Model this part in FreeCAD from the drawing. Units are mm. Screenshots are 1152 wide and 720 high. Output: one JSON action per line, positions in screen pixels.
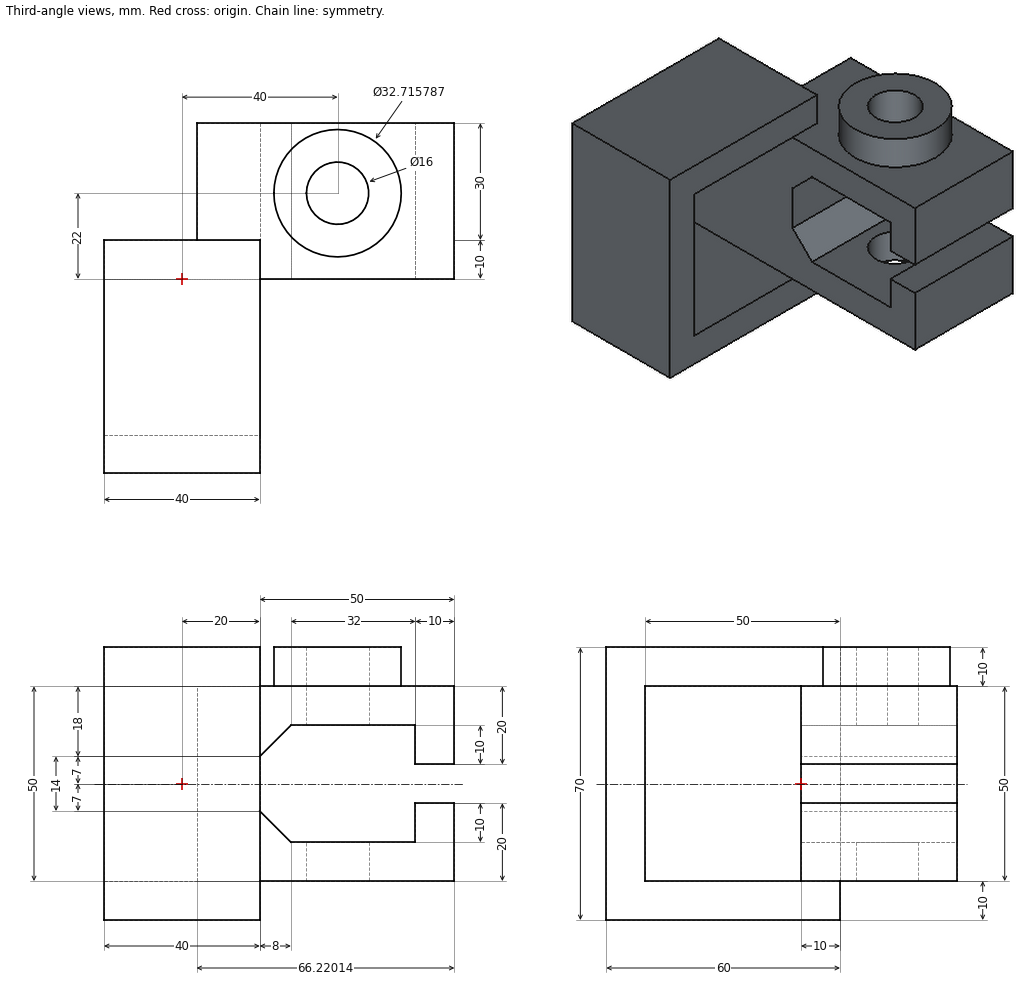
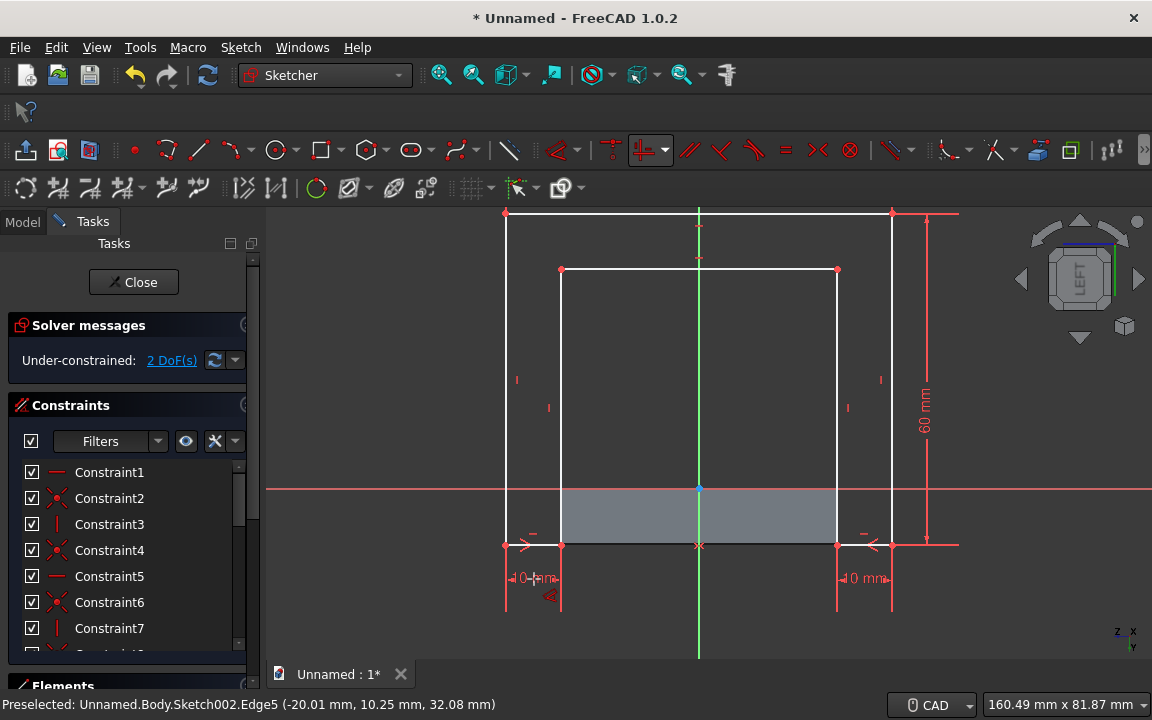
{"action": "left_click", "coordinate": [561, 462]}
{"action": "left_click", "coordinate": [527, 407]}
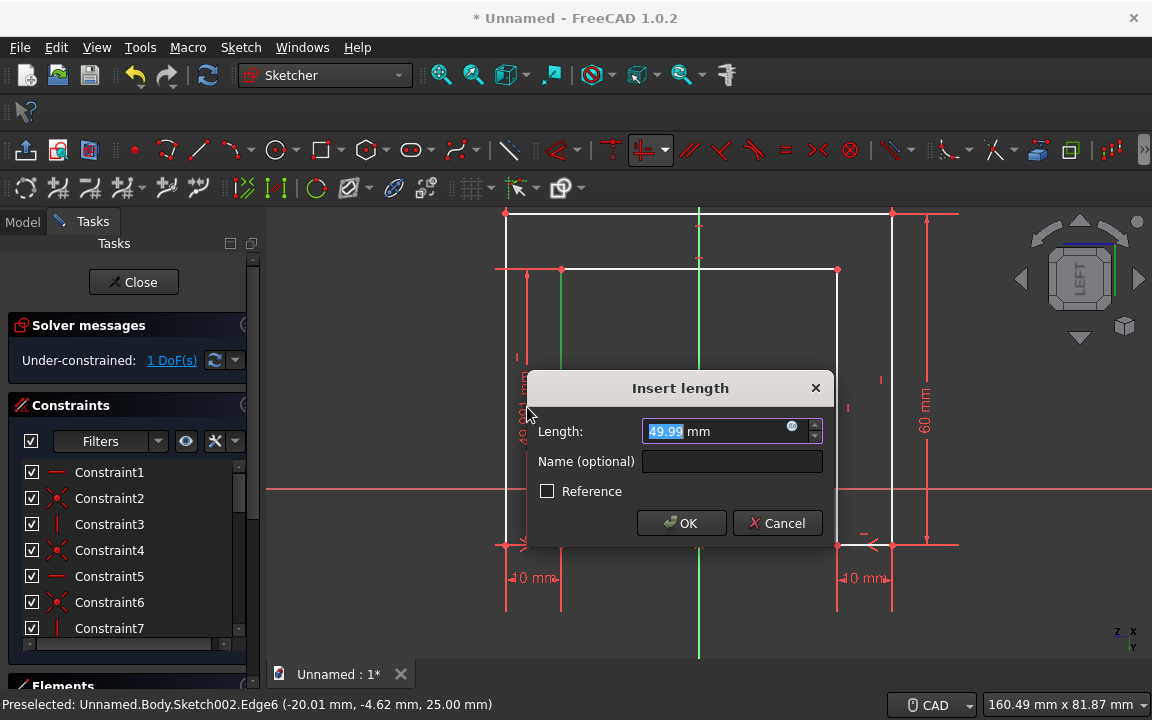
{"action": "type", "text": "50"}
{"action": "key", "text": "Return"}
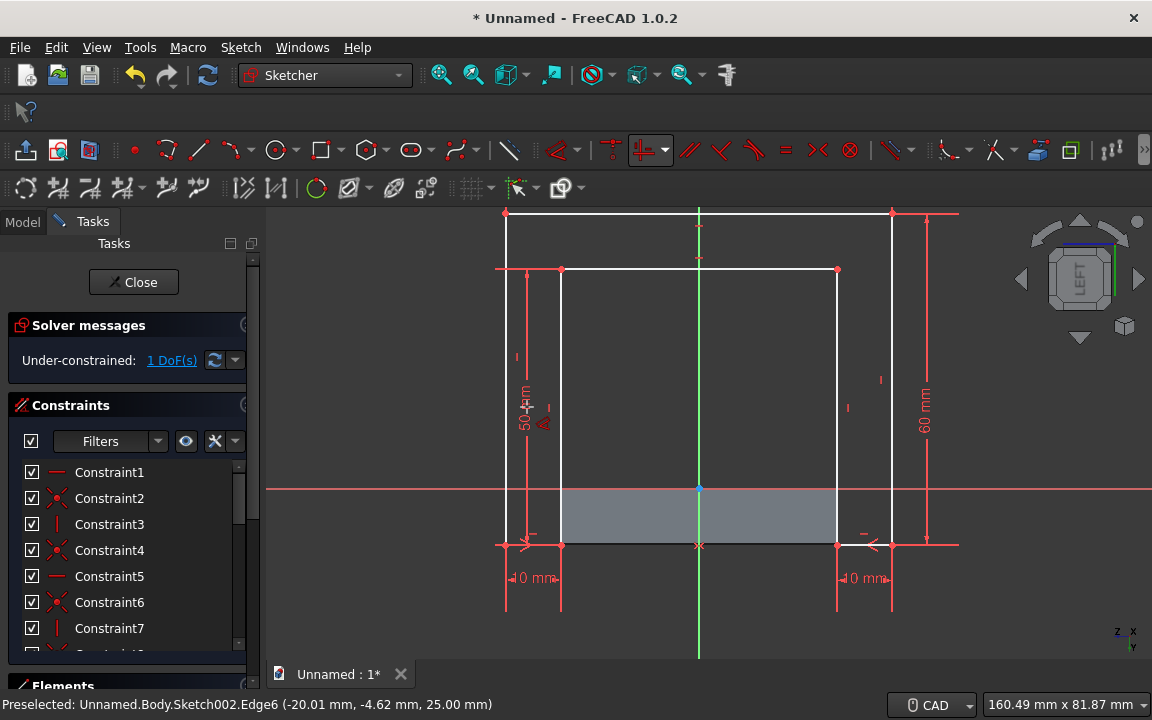
{"action": "left_click", "coordinate": [837, 545]}
{"action": "left_click", "coordinate": [871, 517]}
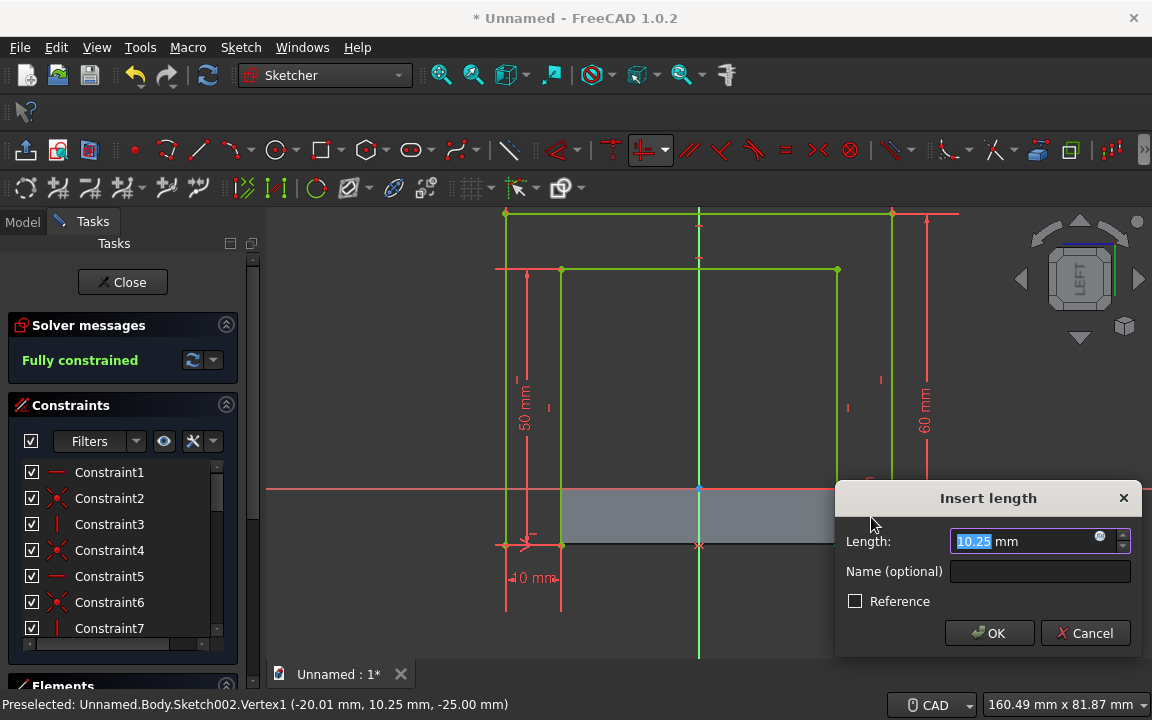
{"action": "type", "text": "10"}
{"action": "key", "text": "Return"}
{"action": "key", "text": "Escape"}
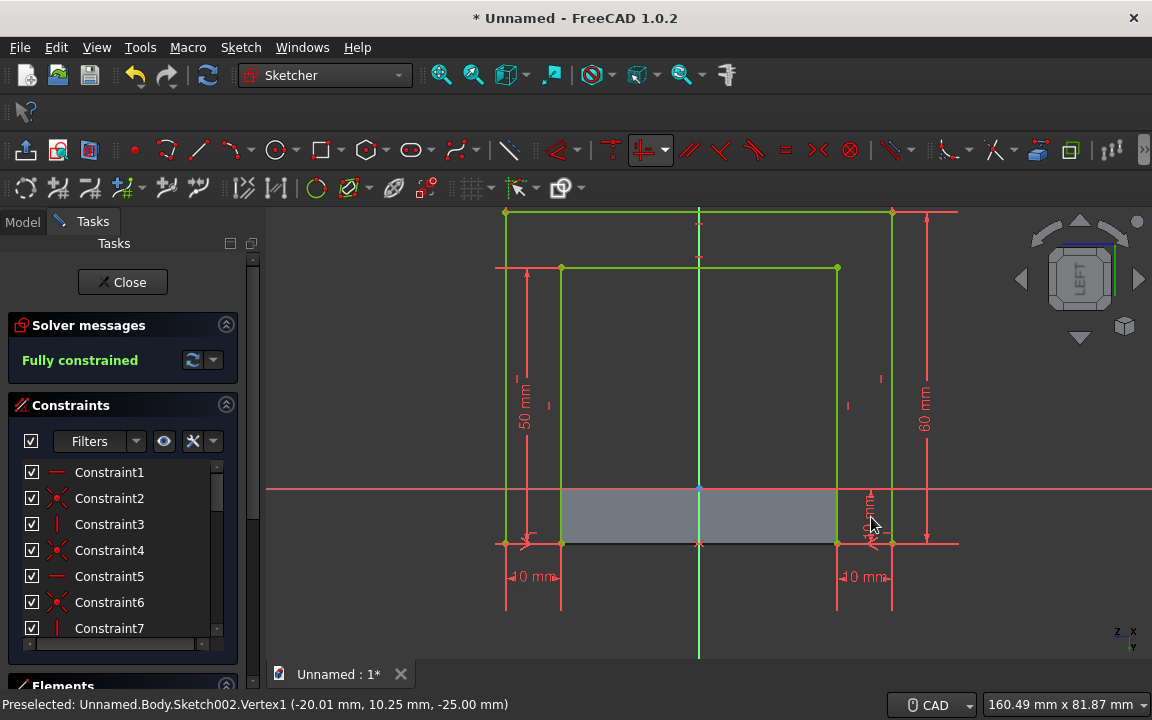
{"action": "left_click", "coordinate": [123, 282]}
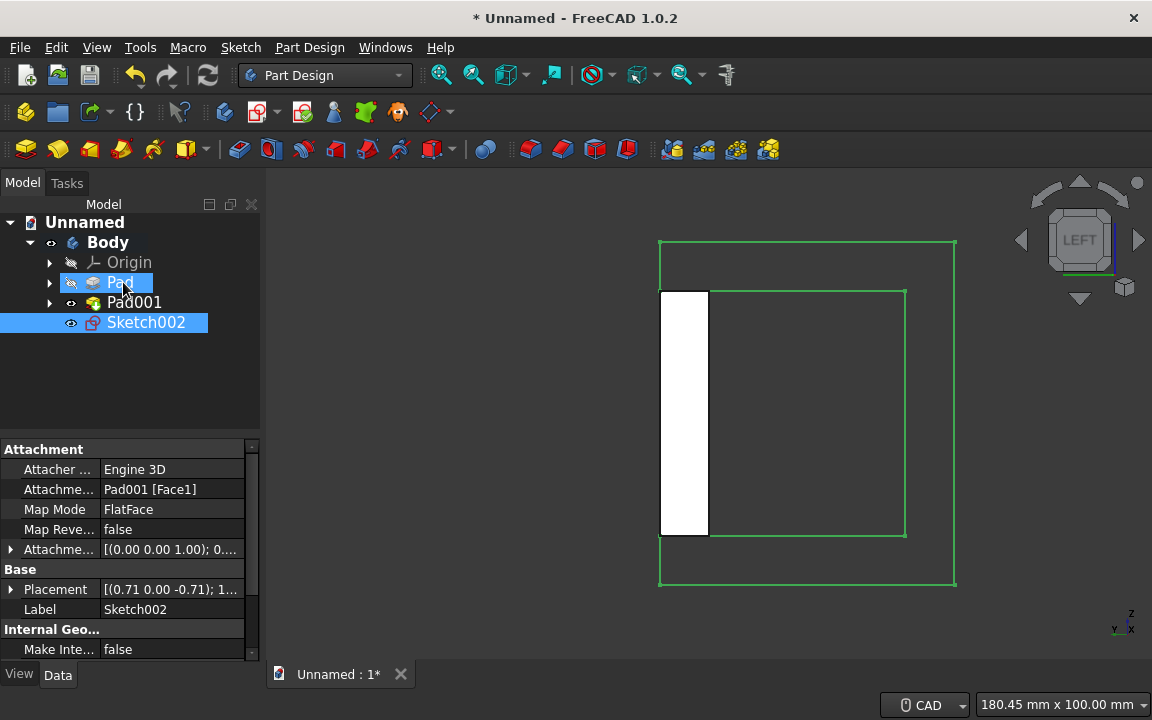
{"action": "left_click", "coordinate": [26, 150]}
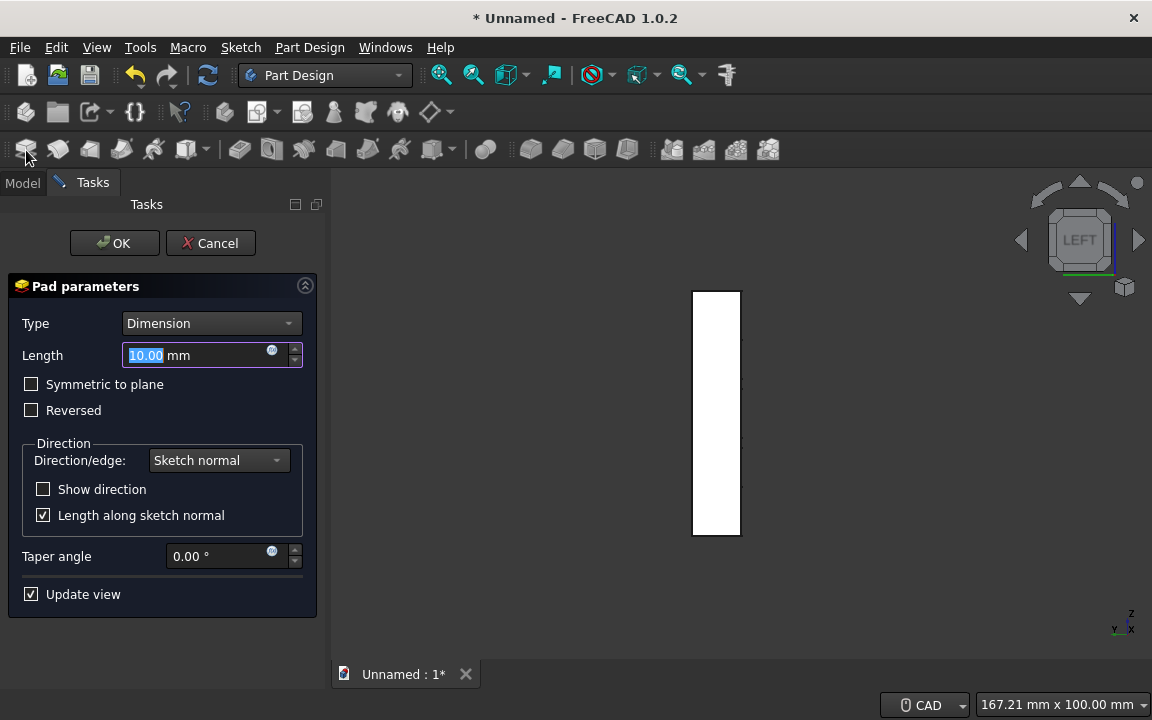
{"action": "type", "text": "40"}
{"action": "key", "text": "Tab"}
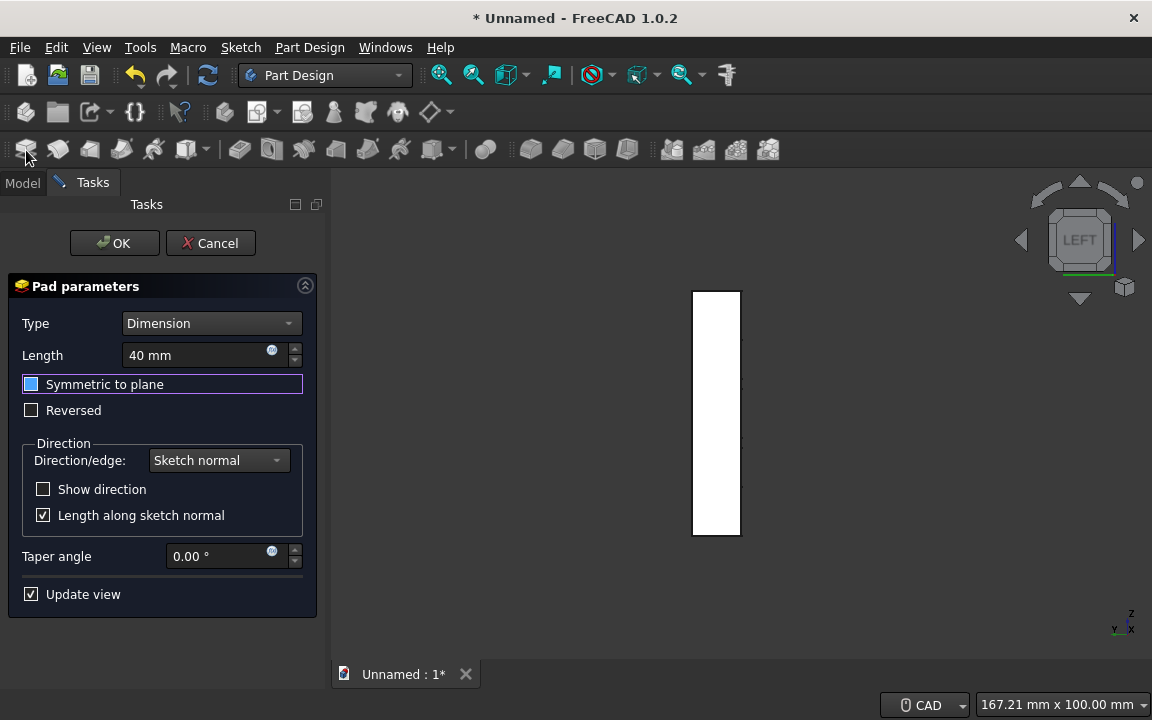
{"action": "left_click", "coordinate": [30, 410]}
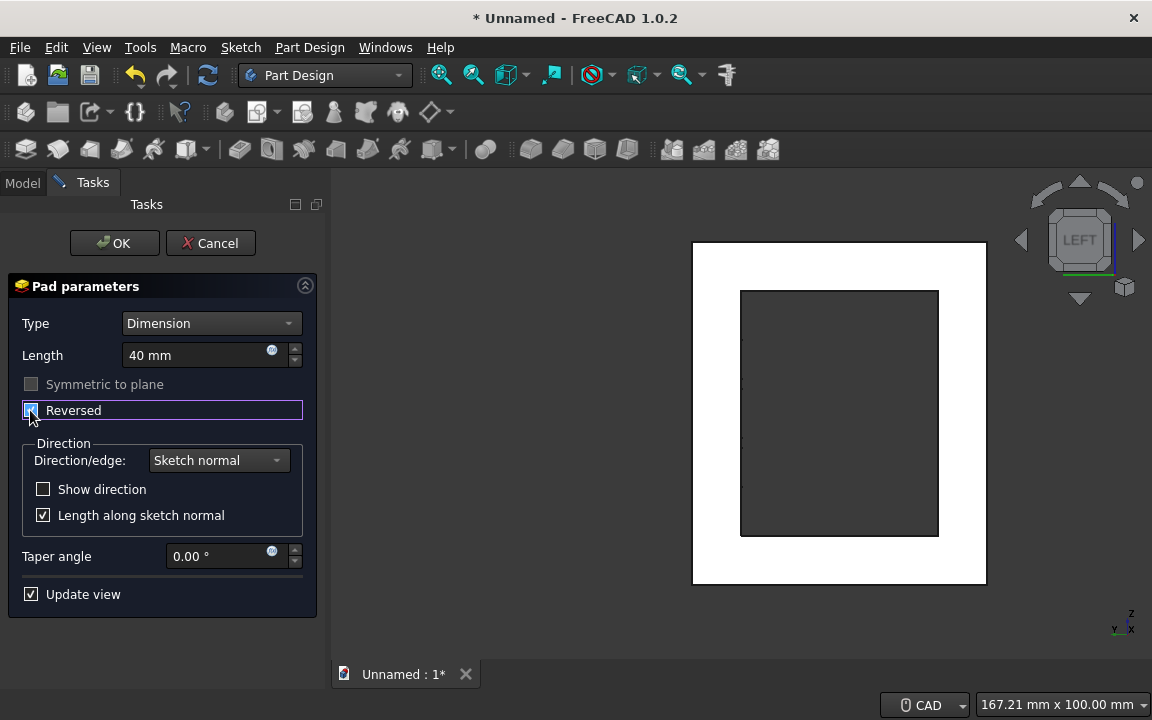
{"action": "left_click", "coordinate": [115, 243]}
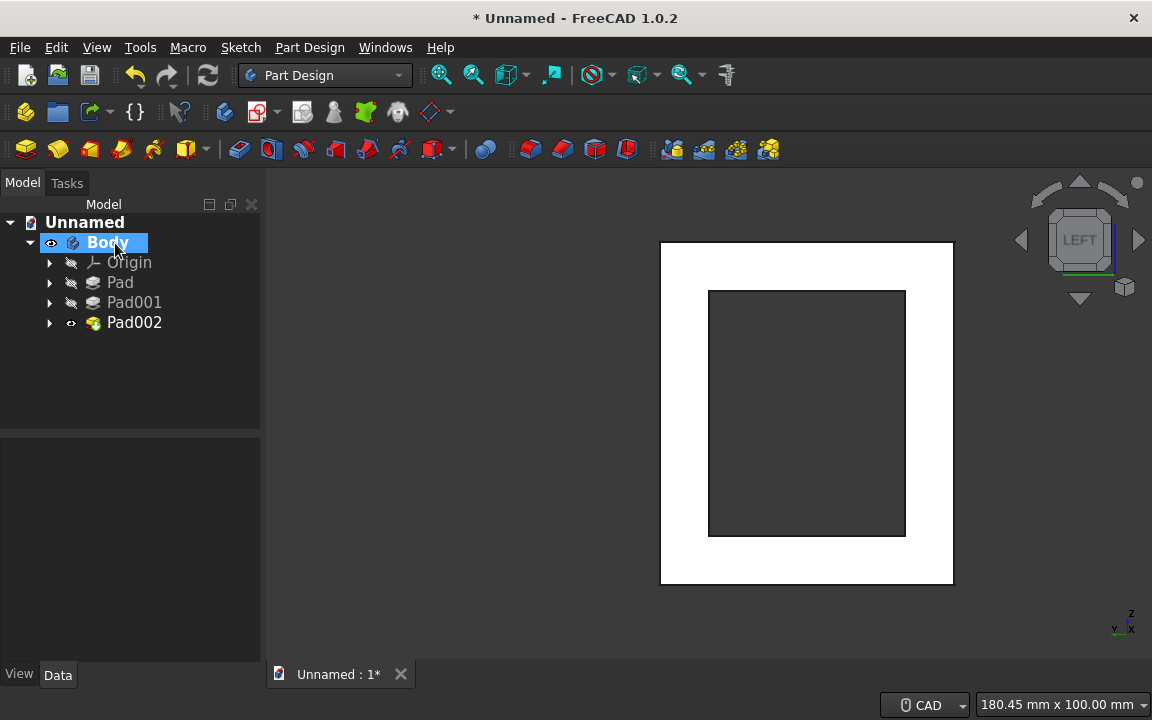
{"action": "key", "text": "4"}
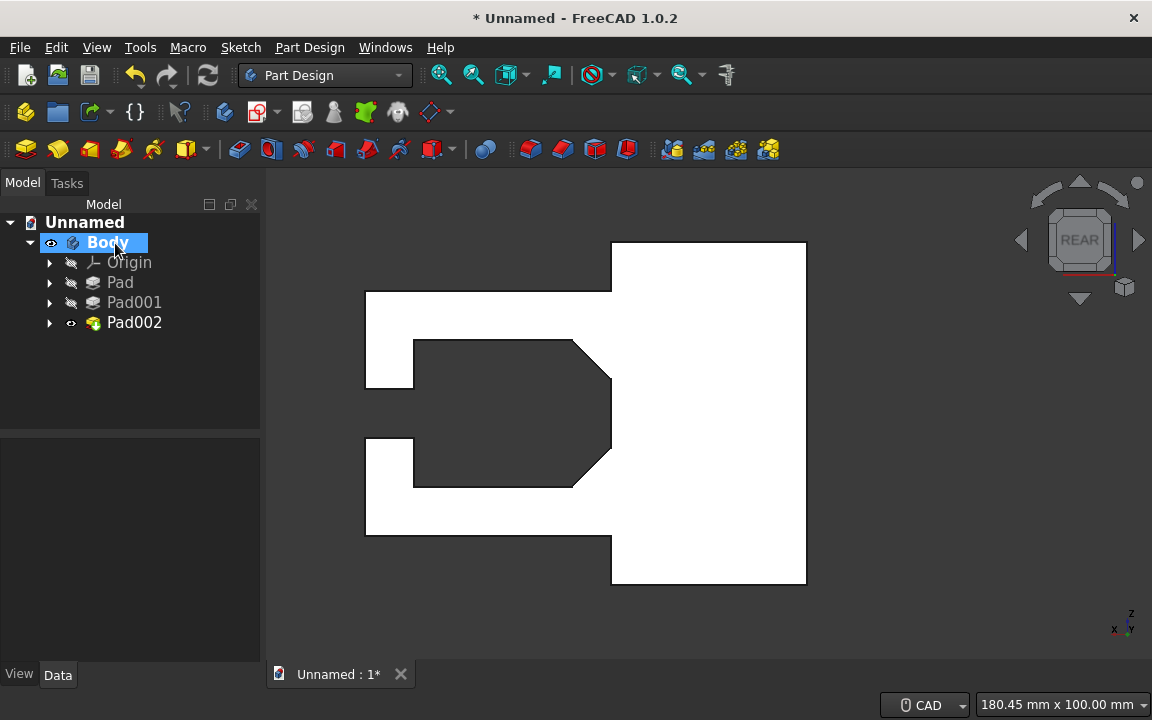
{"action": "left_click", "coordinate": [713, 363]}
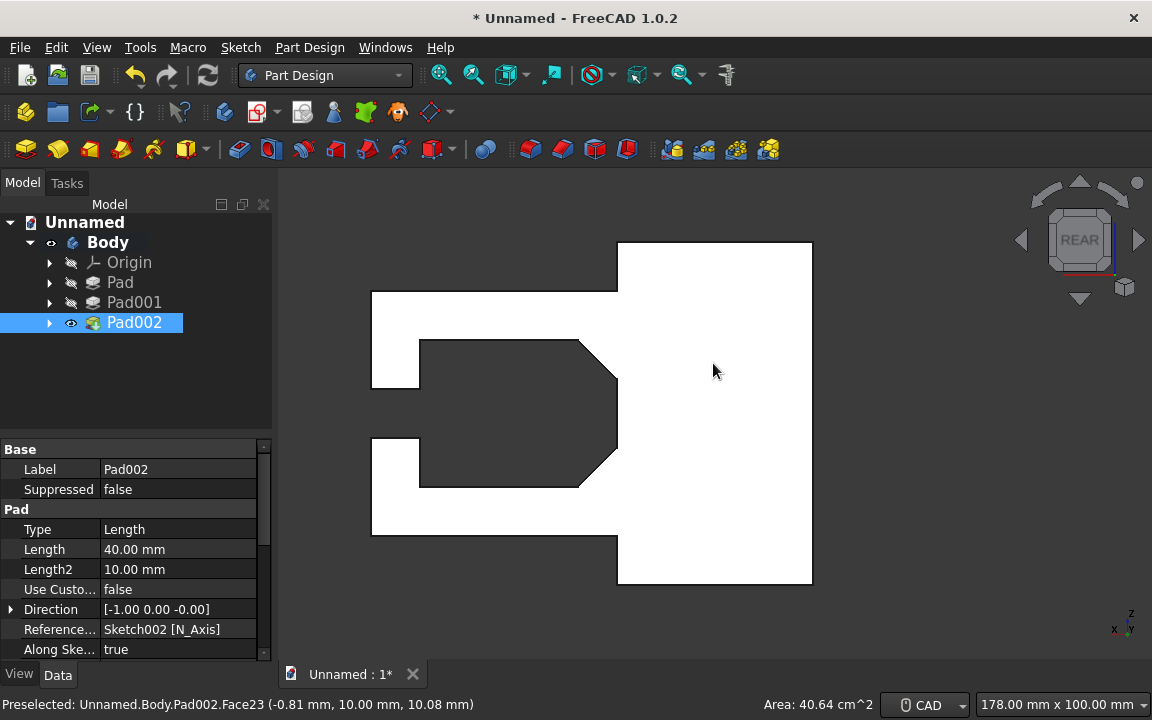
{"action": "left_click", "coordinate": [258, 112]}